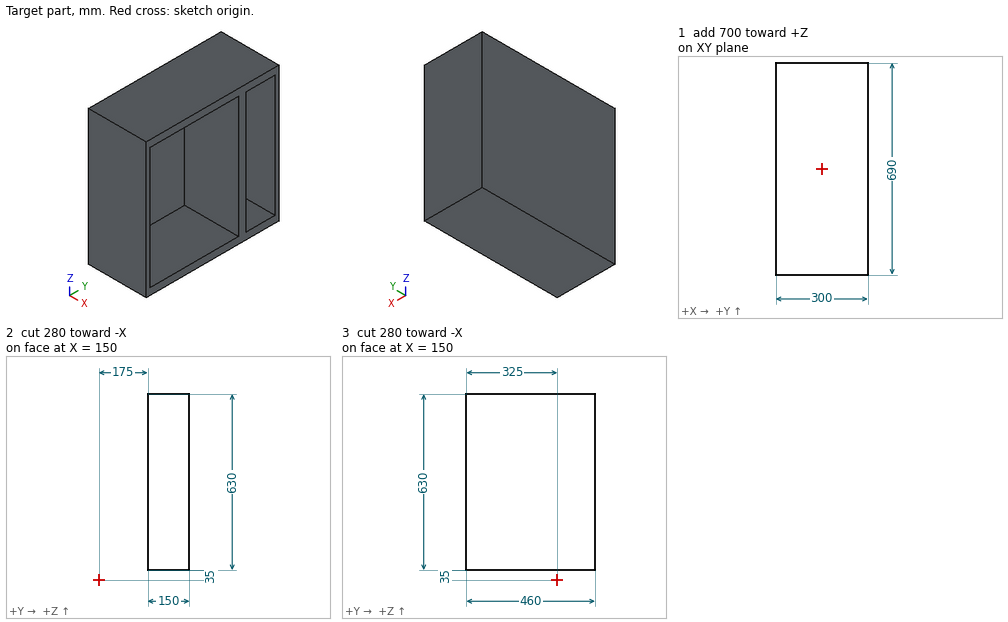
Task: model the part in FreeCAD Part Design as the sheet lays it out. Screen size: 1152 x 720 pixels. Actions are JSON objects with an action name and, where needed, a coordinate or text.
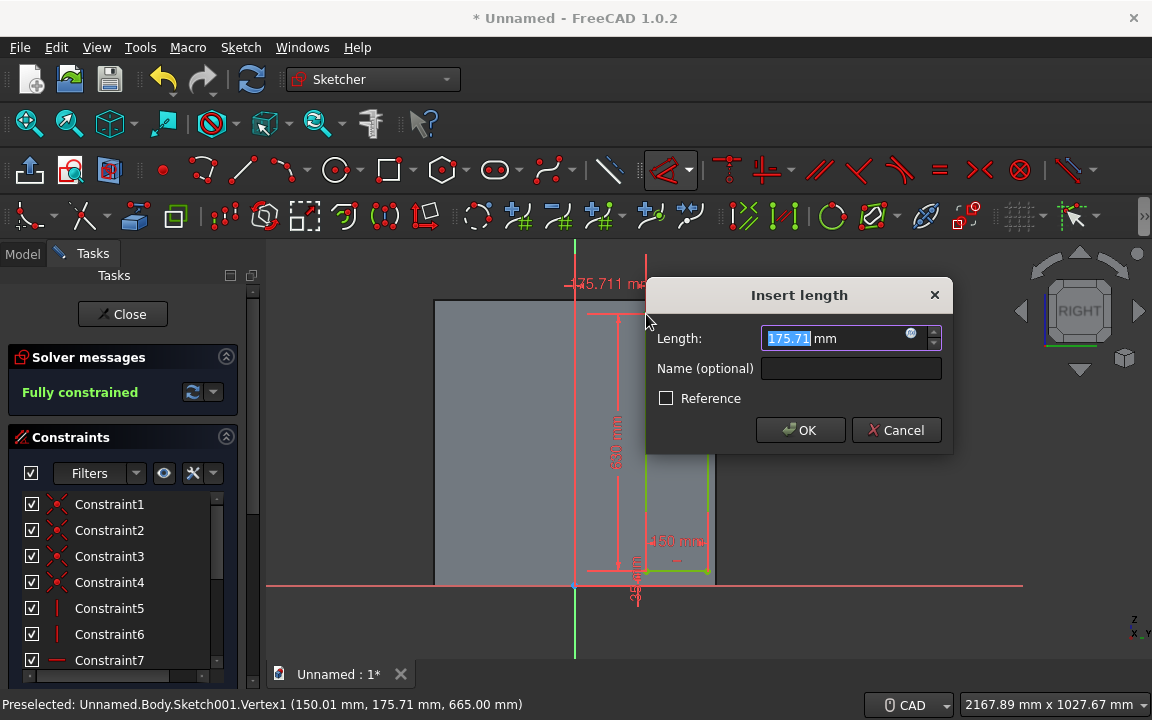
{"action": "type", "text": "175"}
{"action": "key", "text": "Return"}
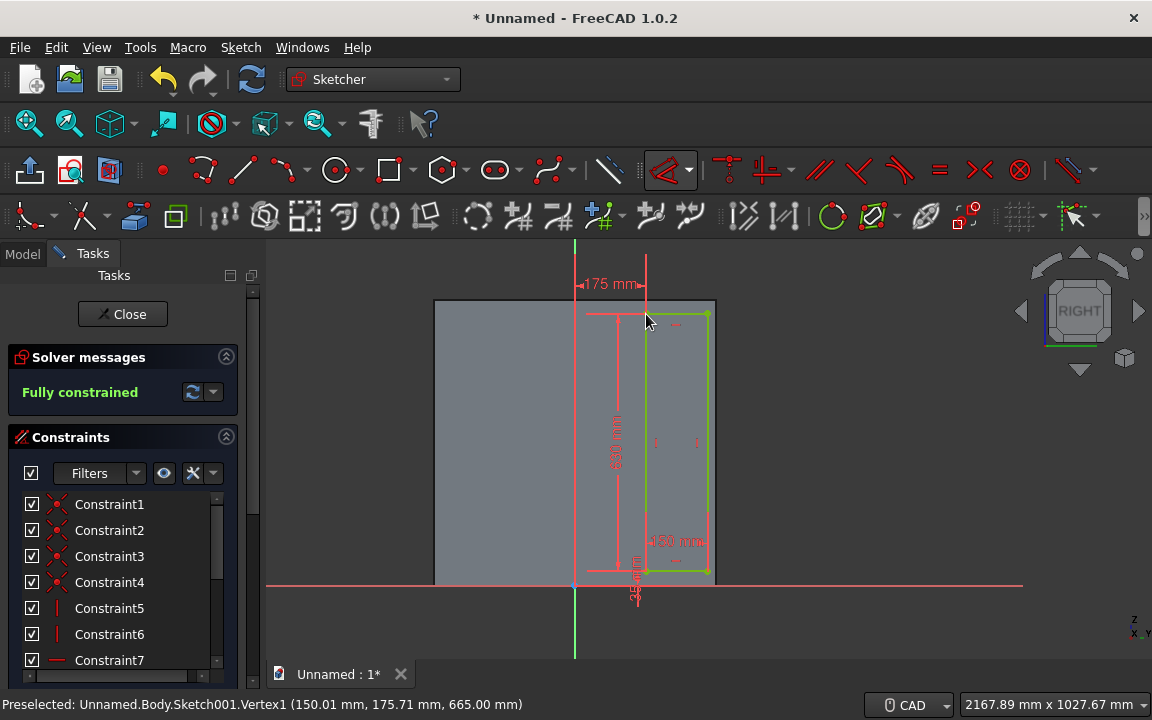
{"action": "left_click", "coordinate": [123, 314]}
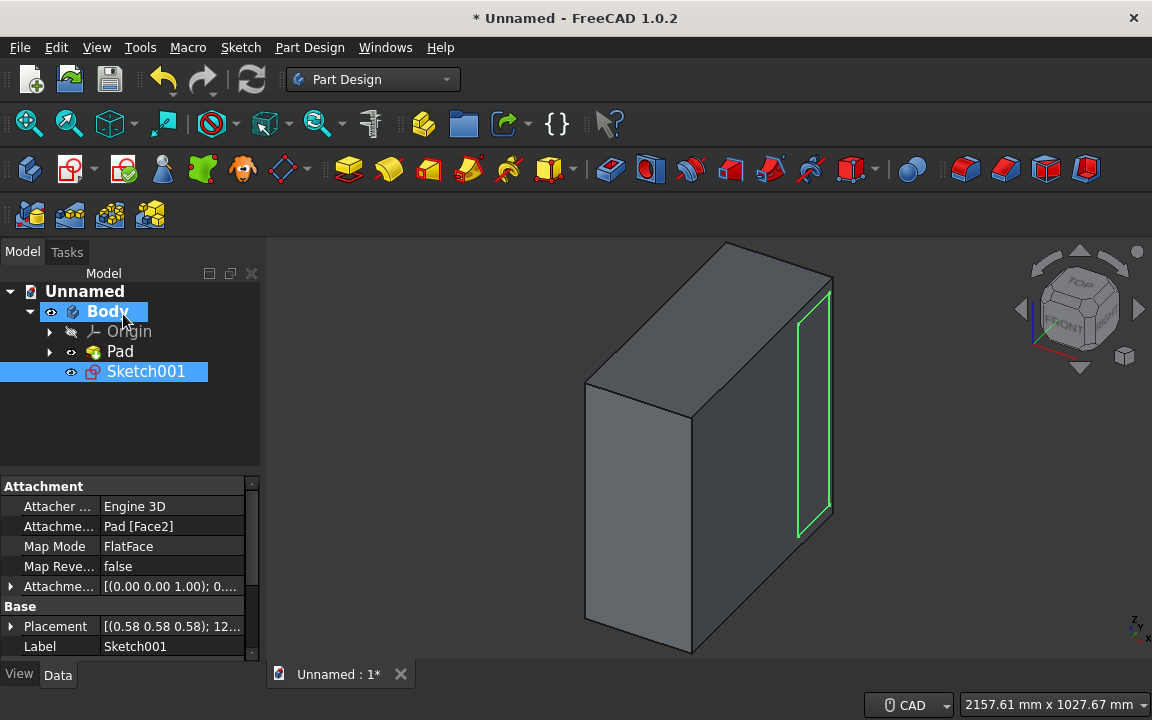
{"action": "left_click", "coordinate": [612, 170]}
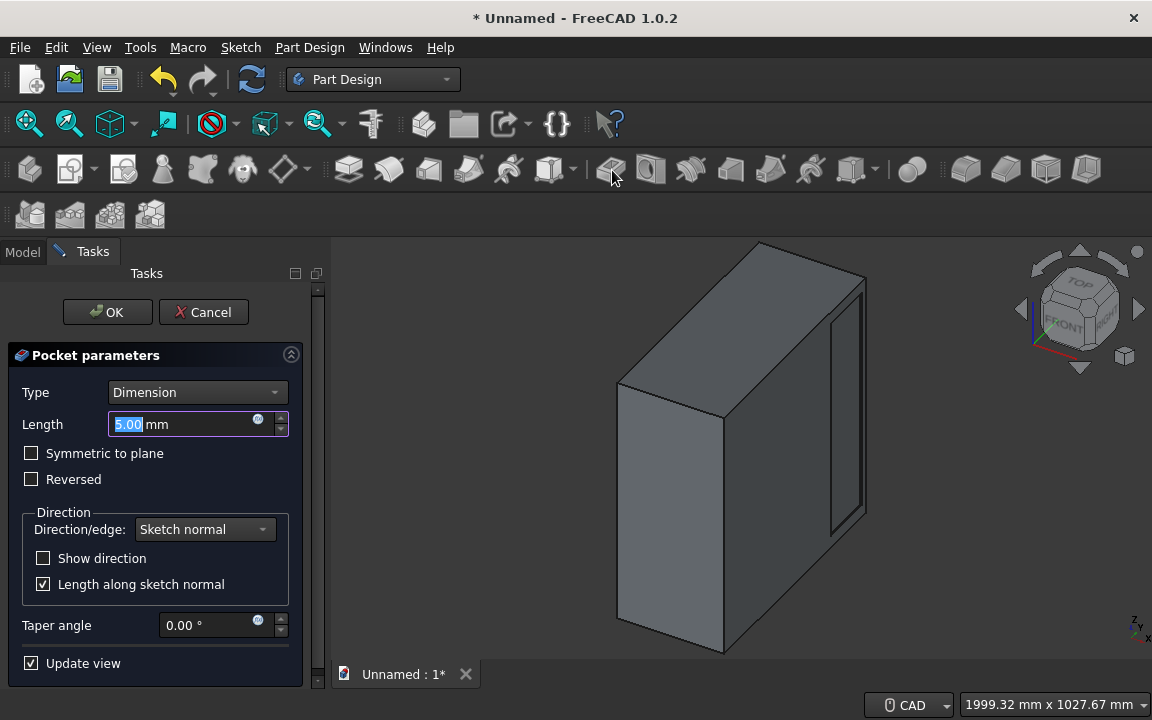
{"action": "type", "text": "280"}
{"action": "key", "text": "Tab"}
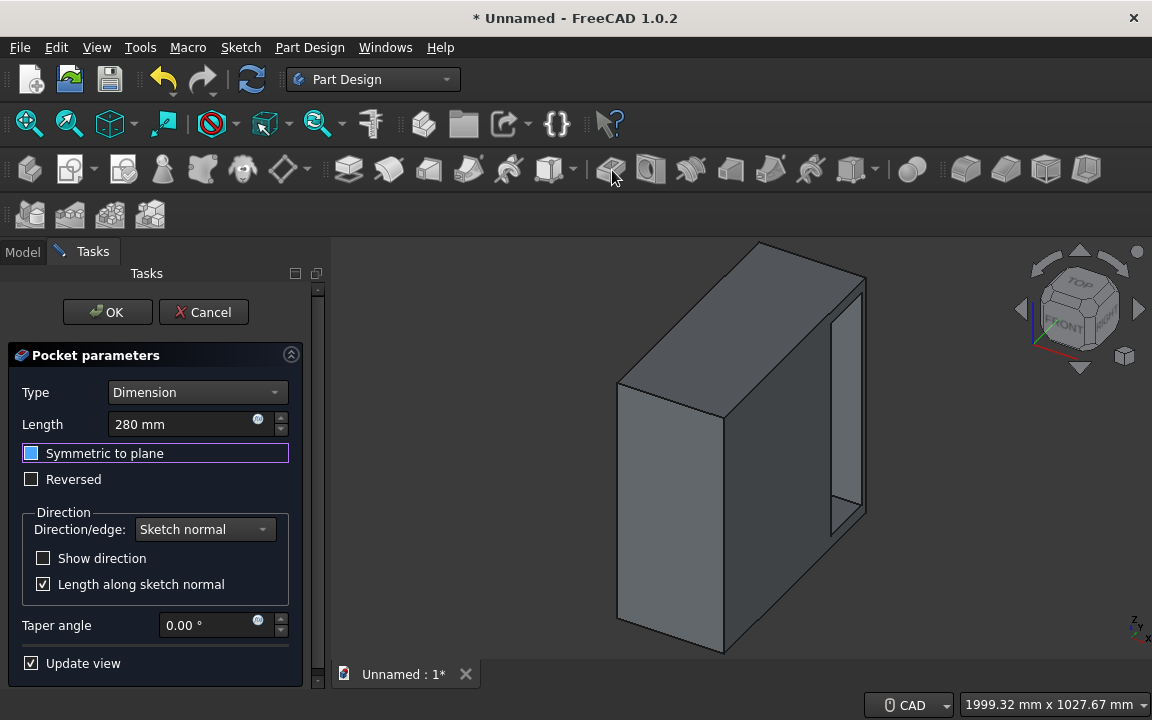
{"action": "left_click", "coordinate": [108, 312]}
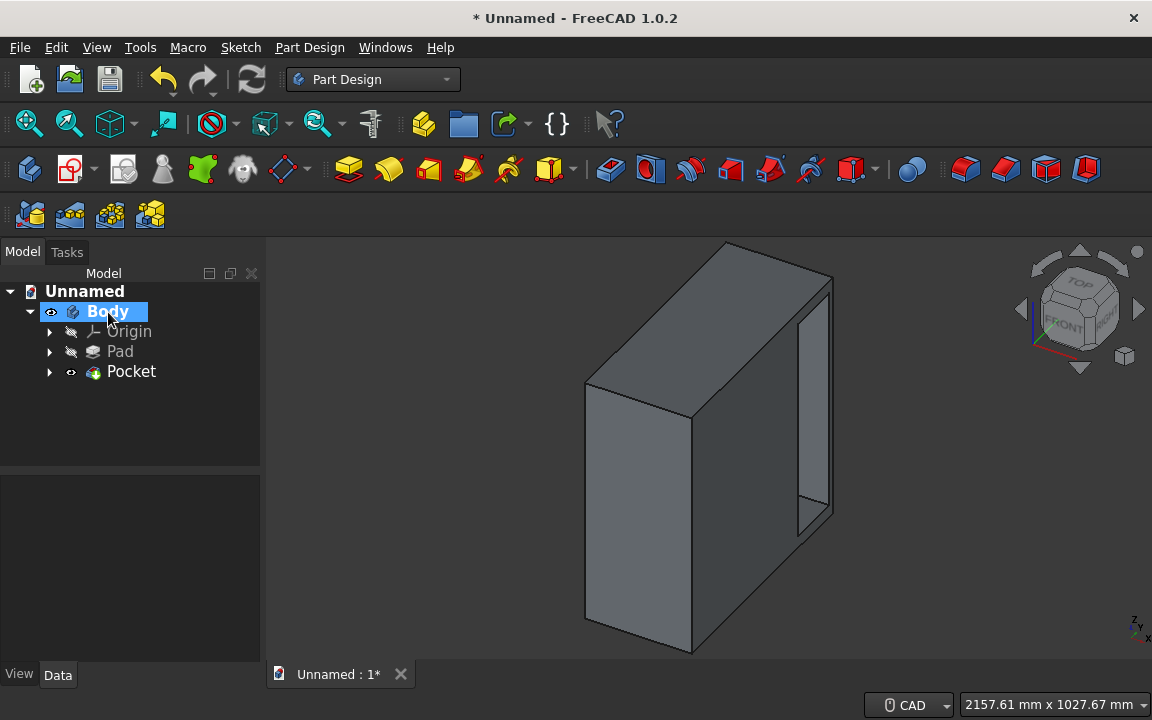
{"action": "left_click", "coordinate": [742, 451]}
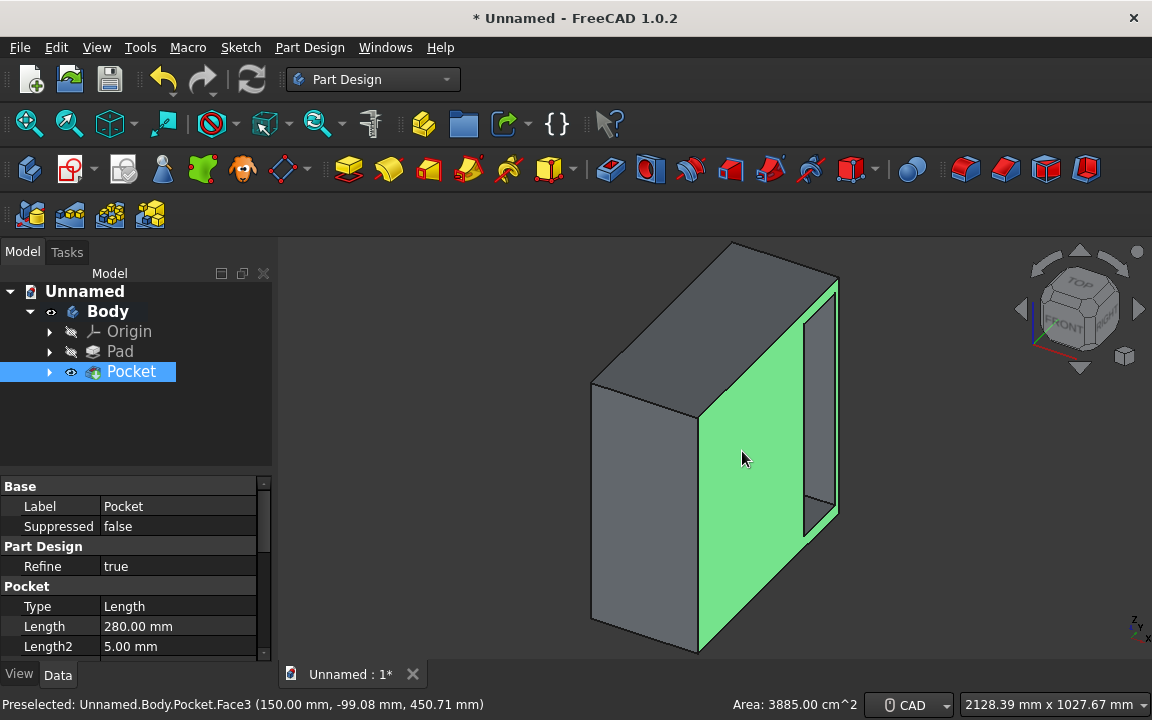
{"action": "left_click", "coordinate": [70, 170]}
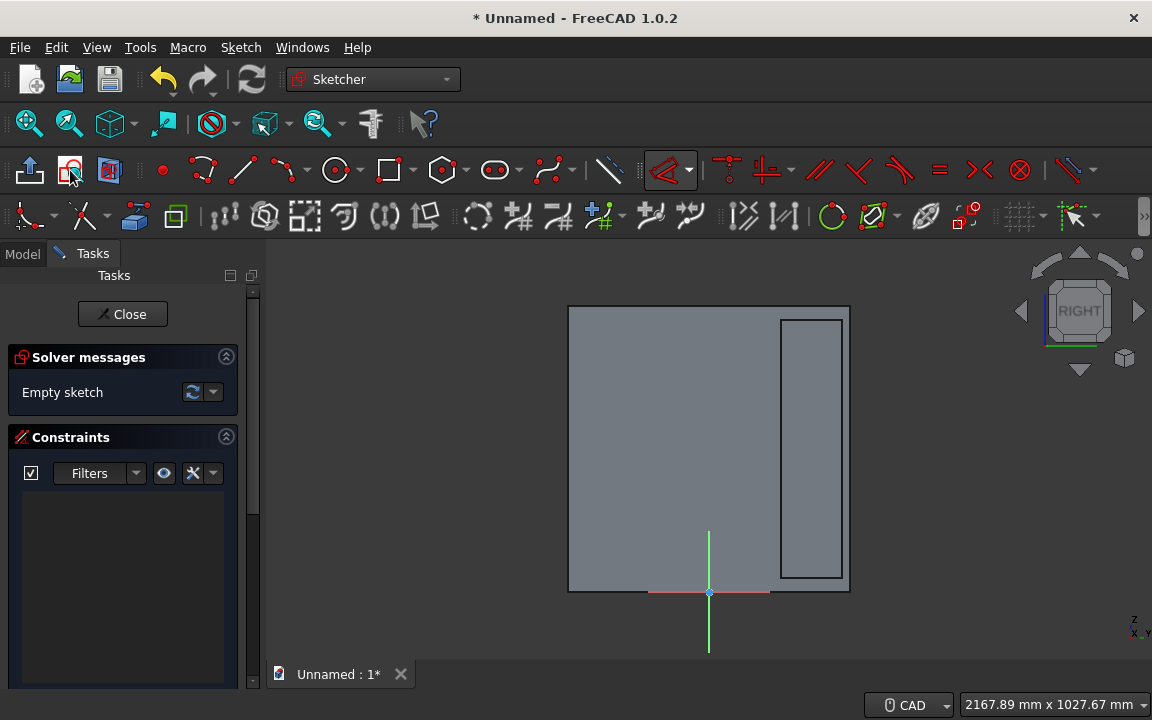
{"action": "key", "text": "g r"}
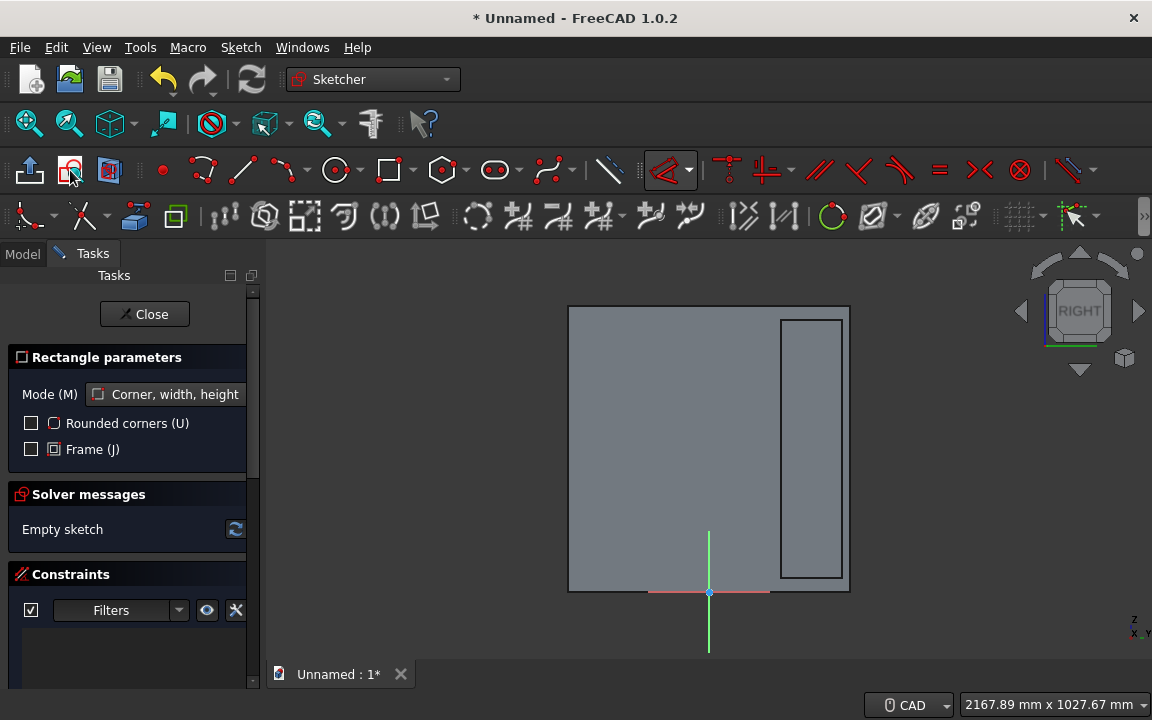
{"action": "left_click", "coordinate": [576, 320]}
{"action": "left_click", "coordinate": [764, 578]}
{"action": "key", "text": "Escape"}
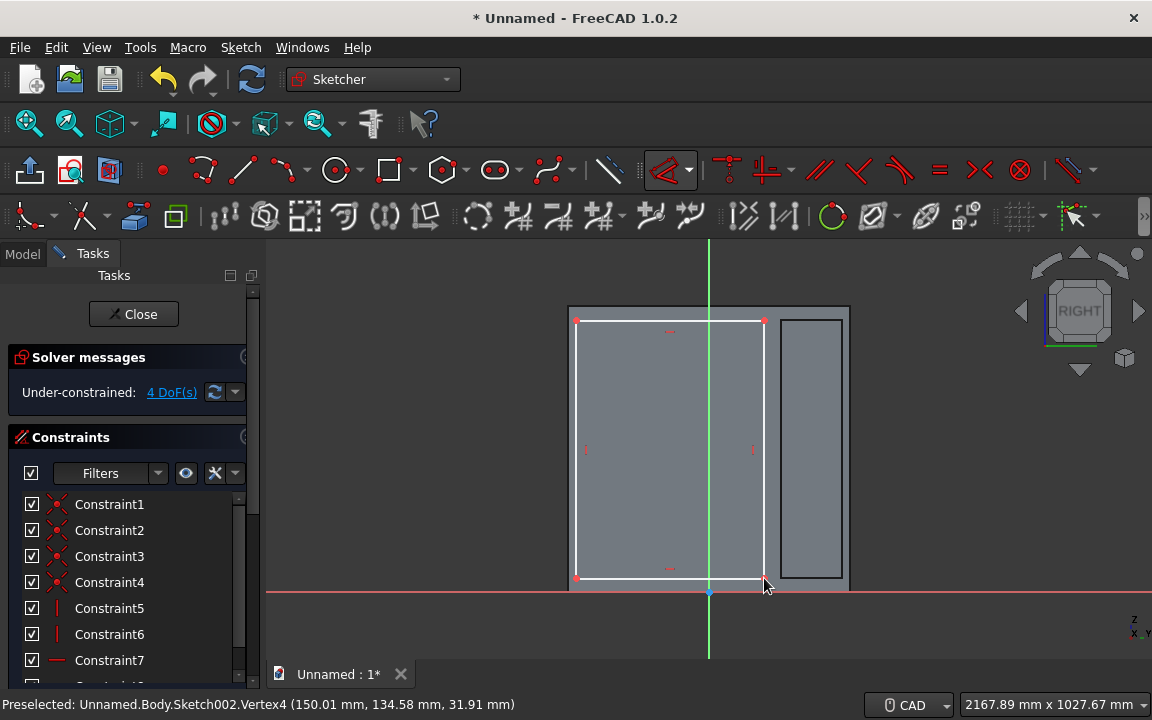
{"action": "left_click", "coordinate": [576, 398]}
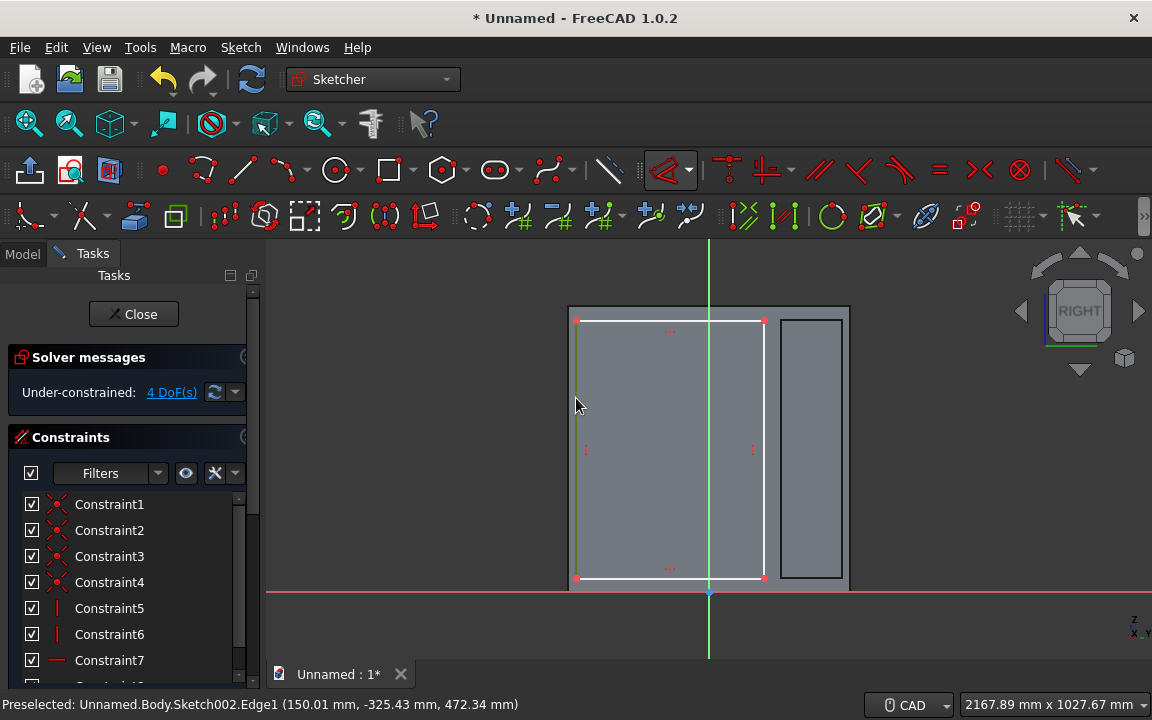
{"action": "key", "text": "i"}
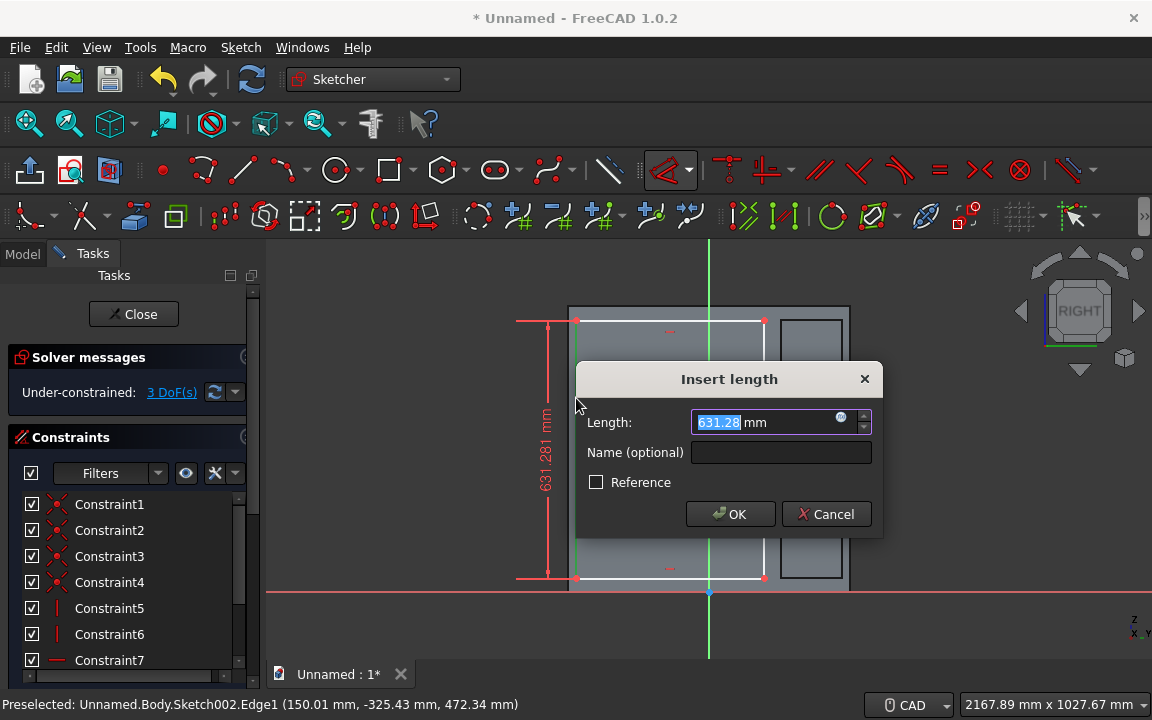
{"action": "type", "text": "630"}
{"action": "key", "text": "Return"}